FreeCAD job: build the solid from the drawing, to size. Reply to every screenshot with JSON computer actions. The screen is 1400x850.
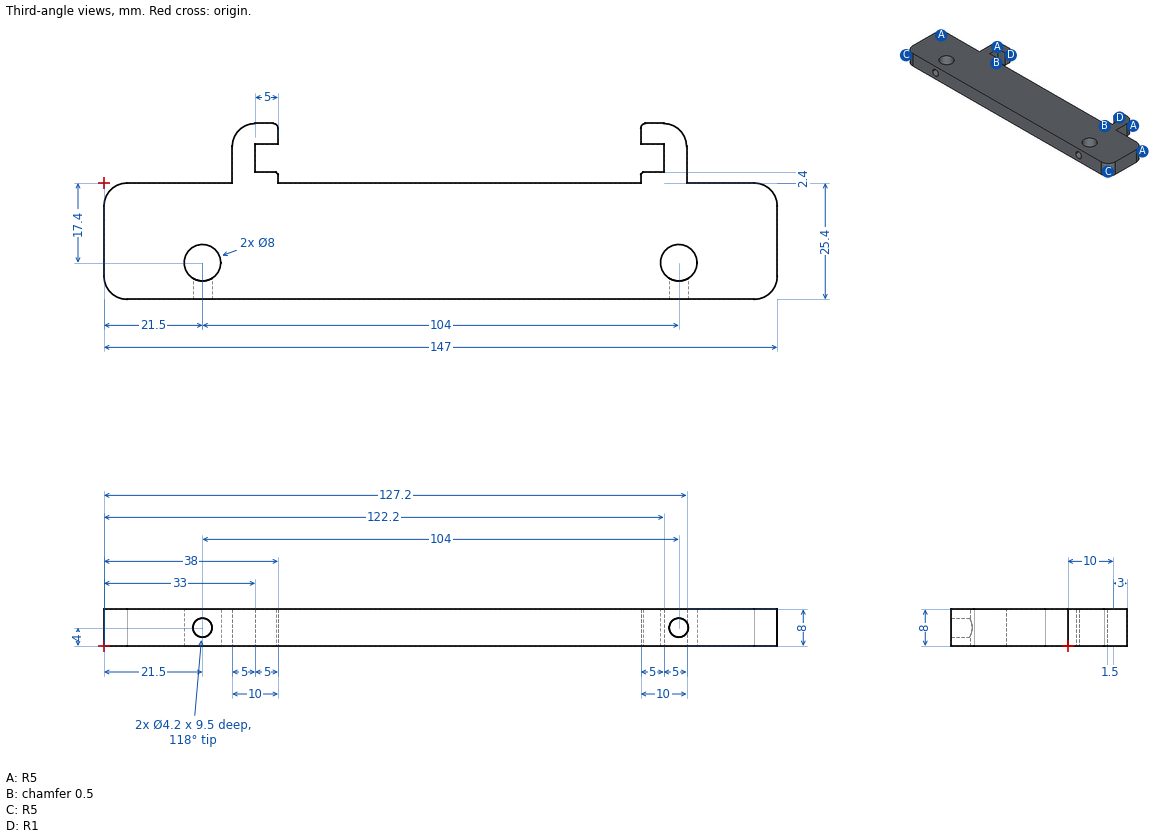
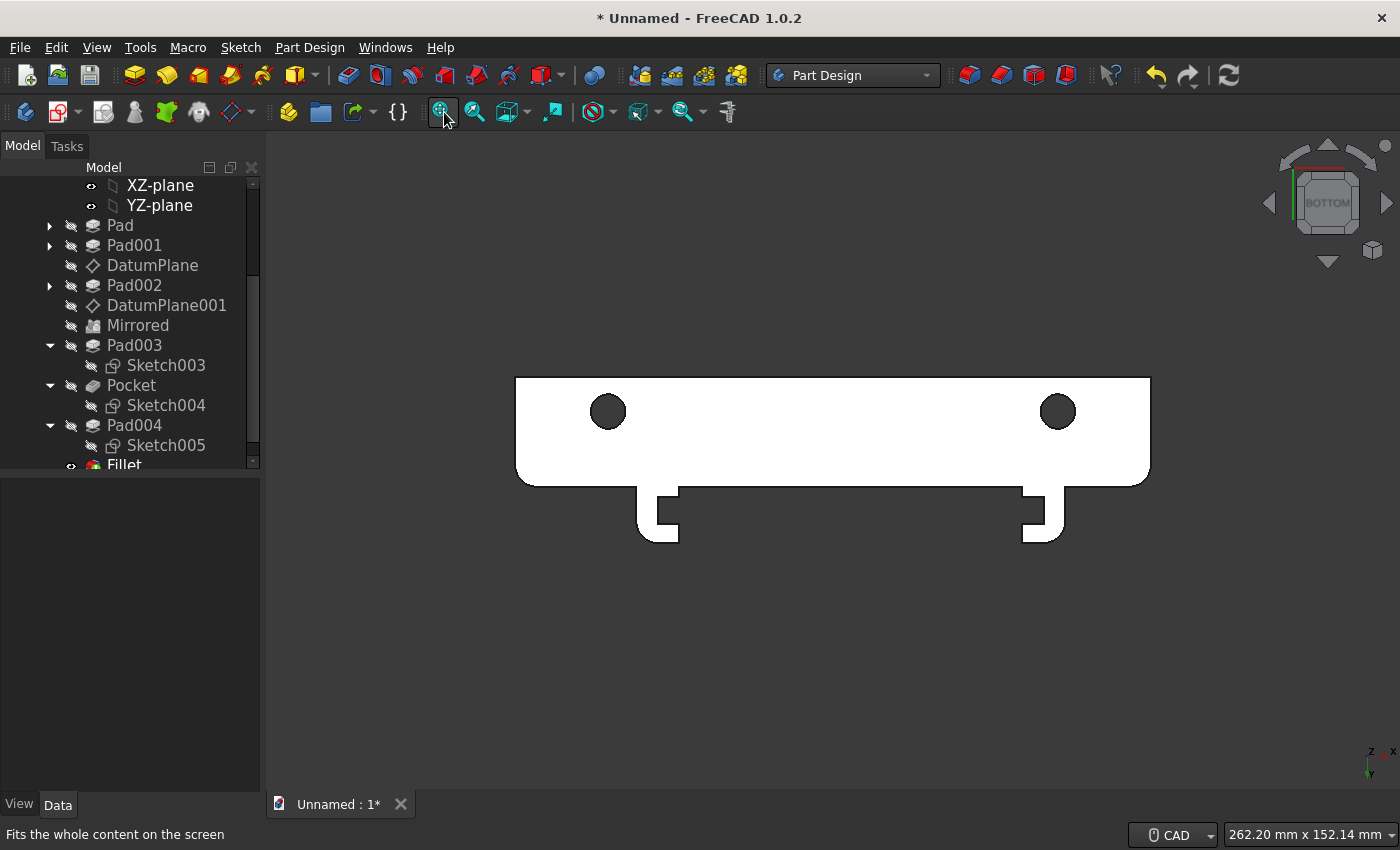
{"action": "key", "text": "4"}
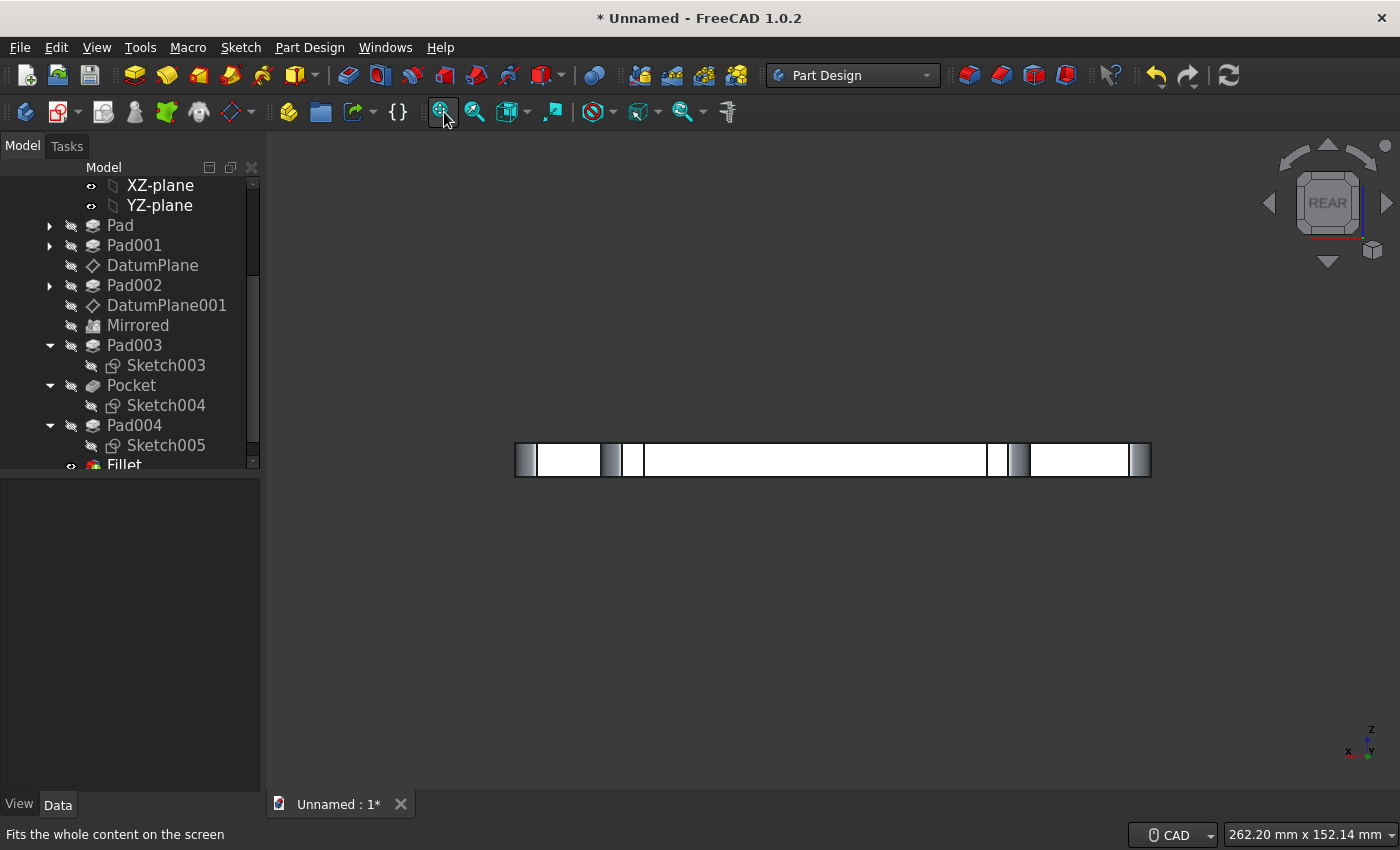
{"action": "key", "text": "6"}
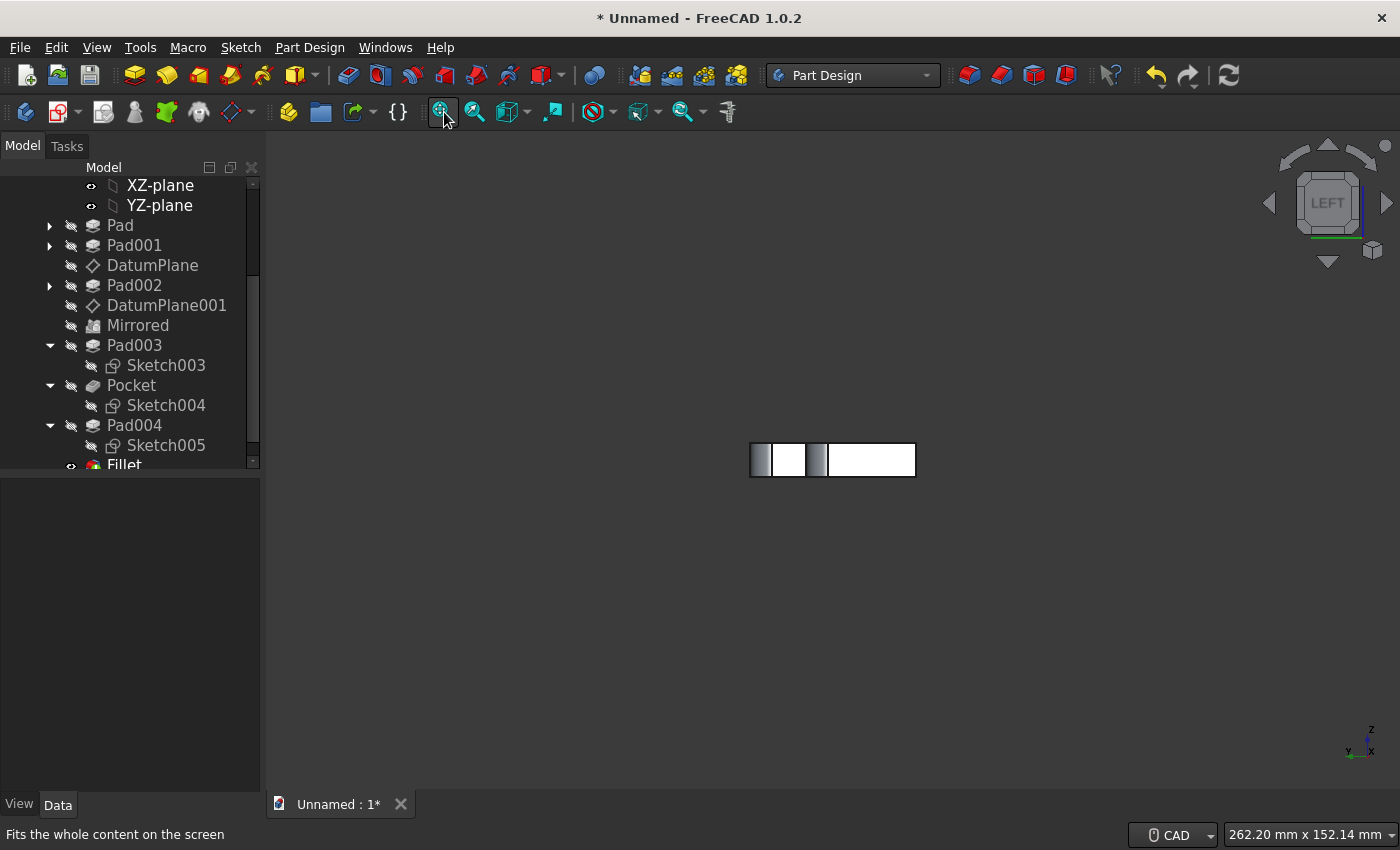
{"action": "key", "text": "v f"}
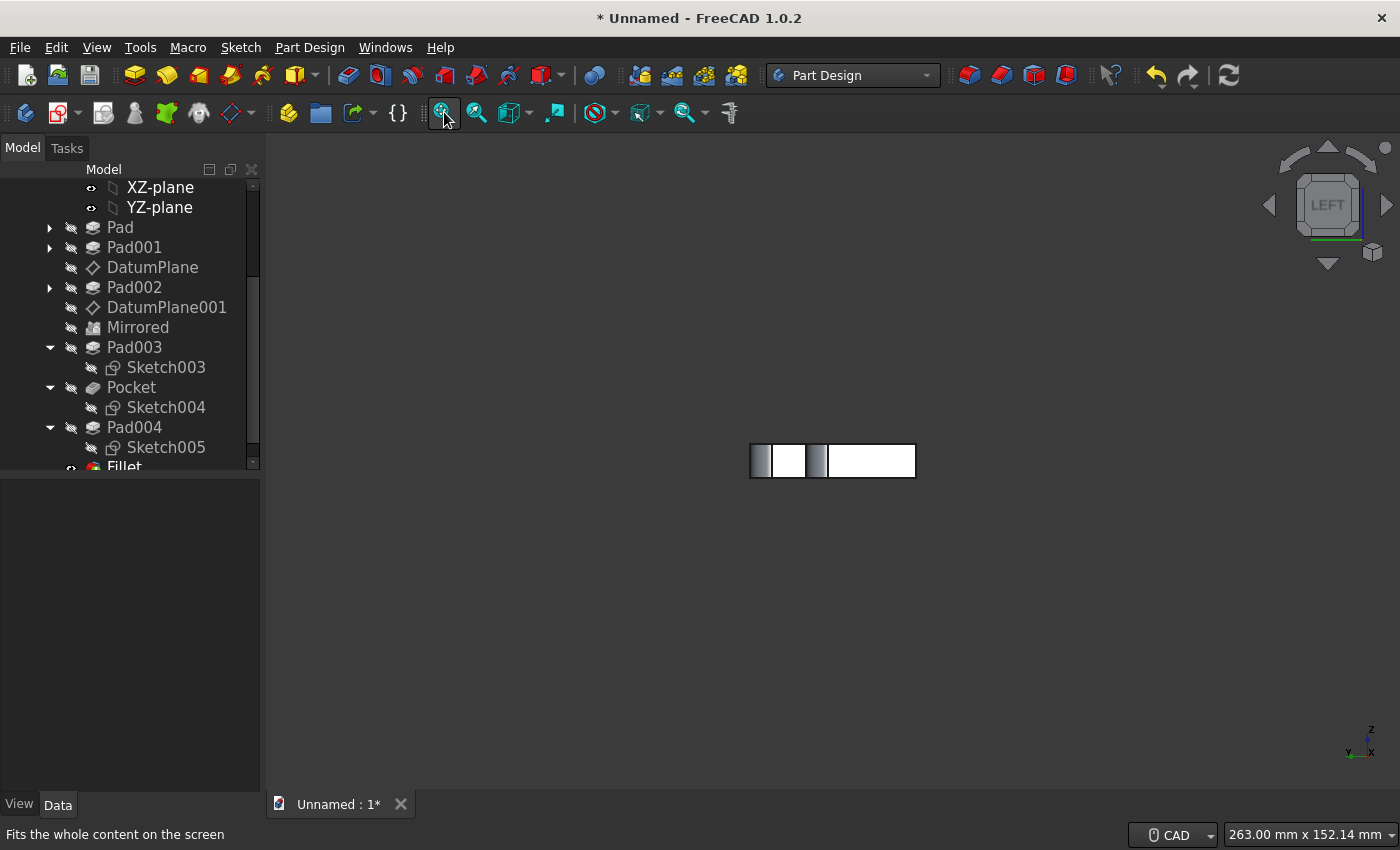
{"action": "key", "text": "v 3"}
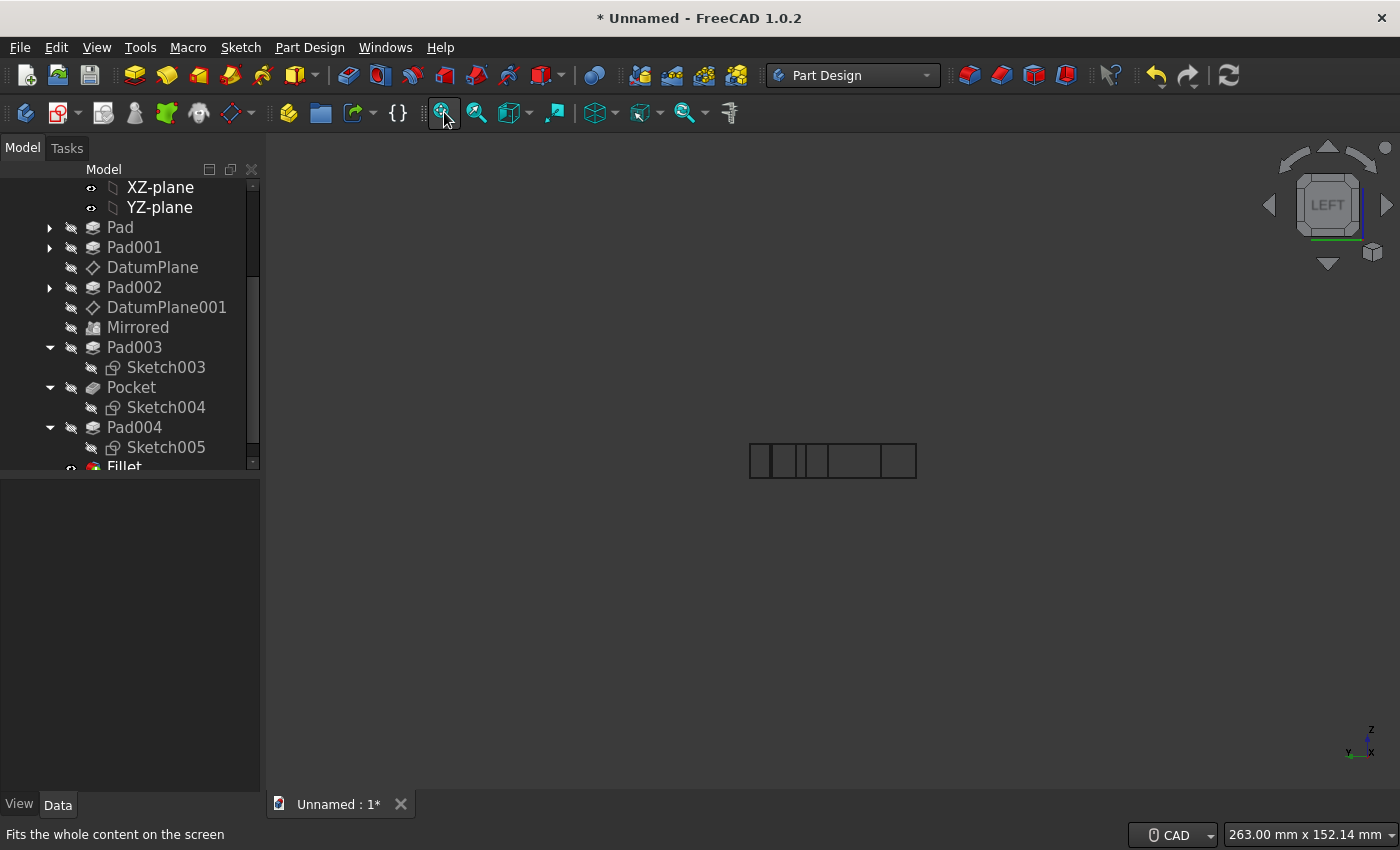
{"action": "key", "text": "0"}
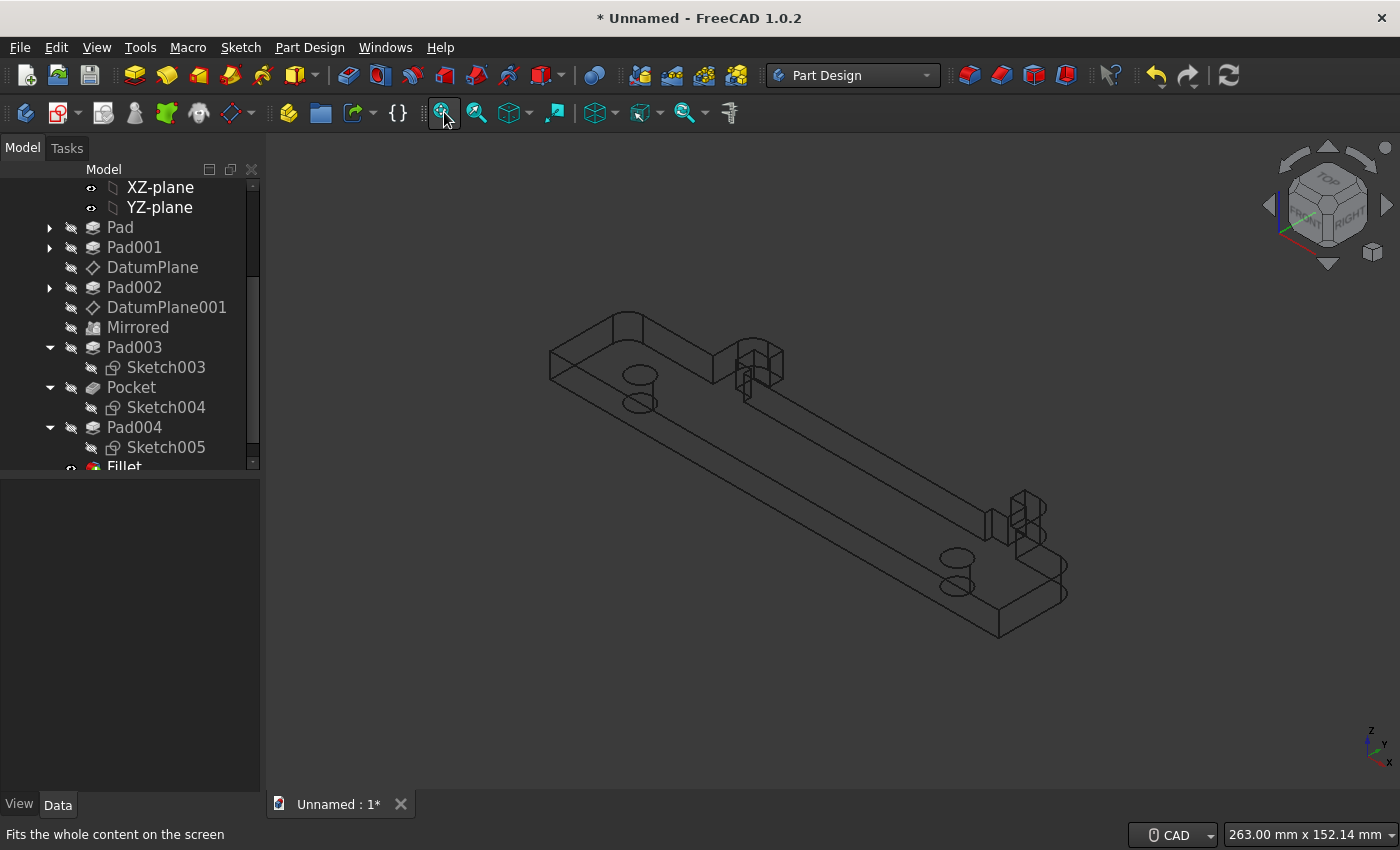
{"action": "left_click", "coordinate": [751, 385]}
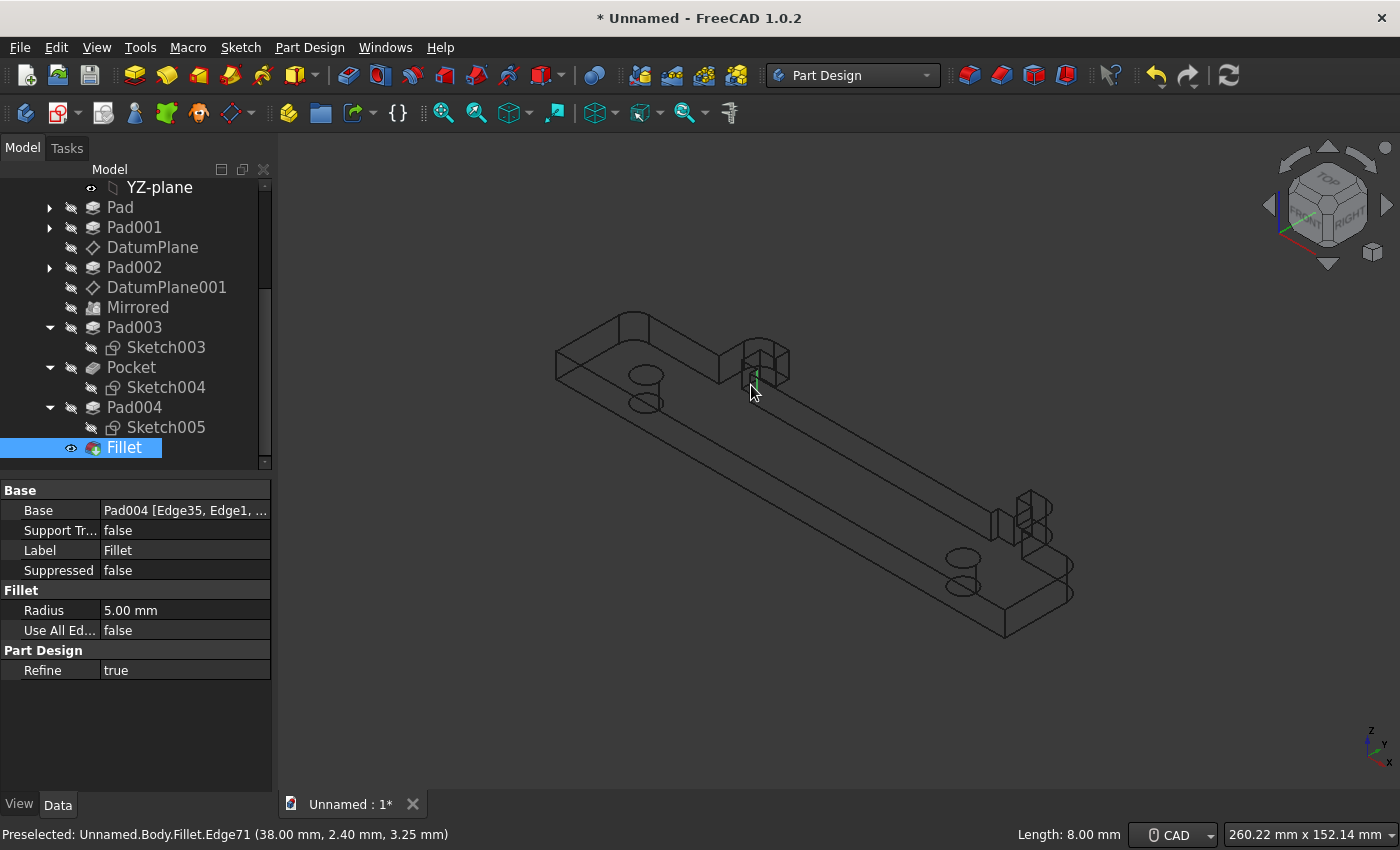
{"action": "left_click", "coordinate": [998, 522], "text": "ctrl"}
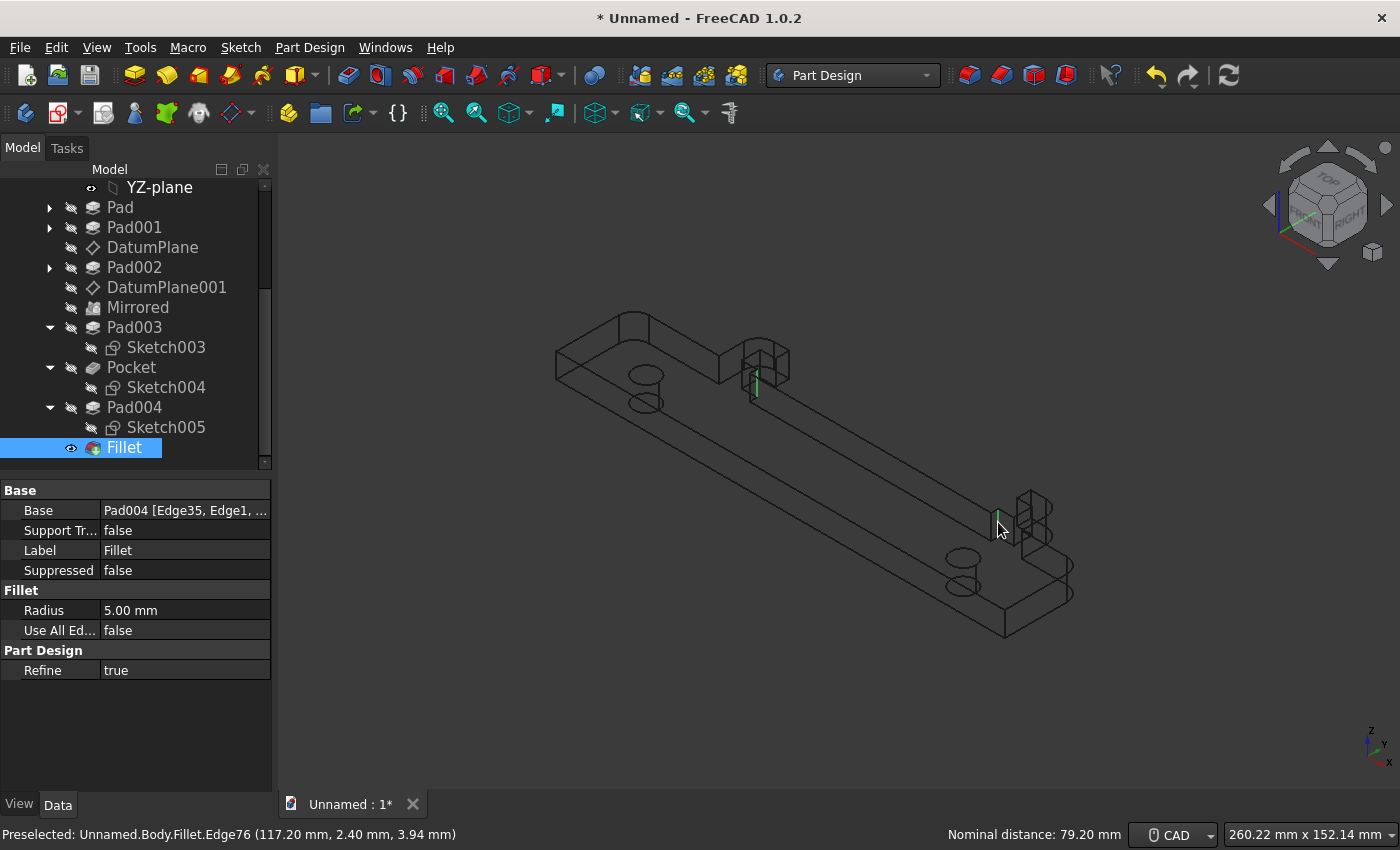
{"action": "key", "text": "v 1"}